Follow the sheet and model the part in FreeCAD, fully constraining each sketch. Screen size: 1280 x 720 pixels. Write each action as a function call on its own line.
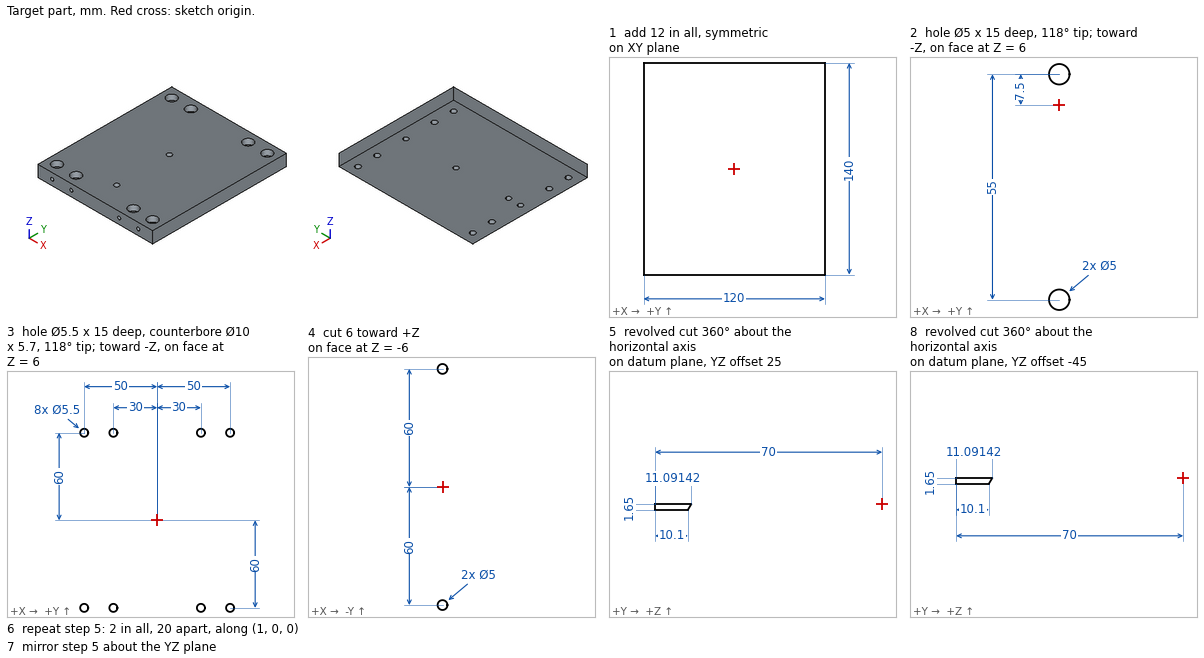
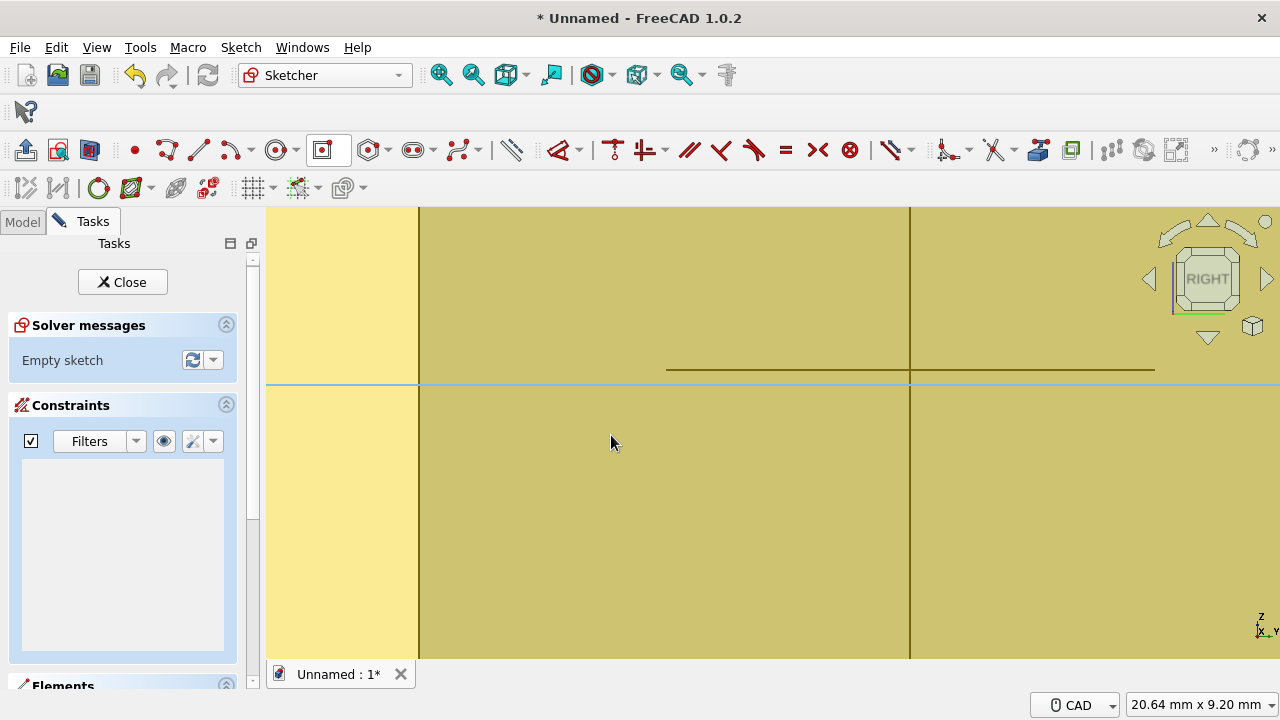
key(g)
key(m)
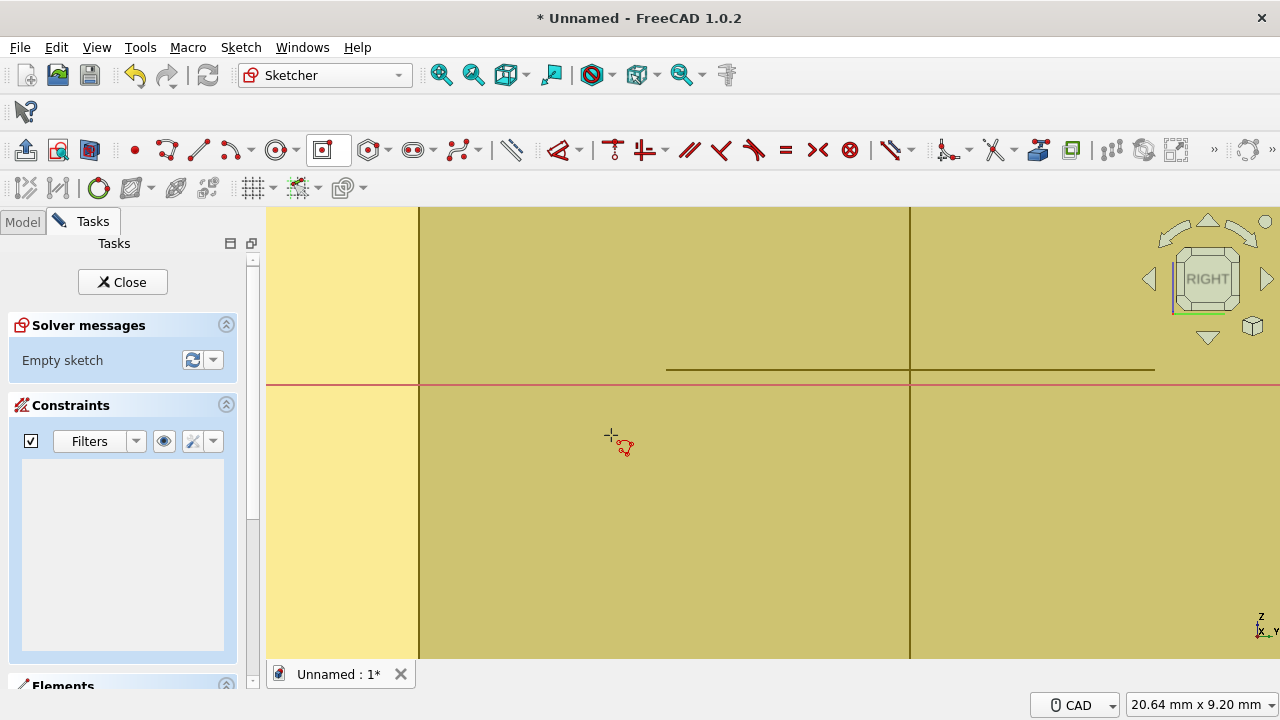
click(964, 385)
click(915, 466)
click(419, 466)
click(419, 394)
click(964, 385)
key(Escape)
key(Escape)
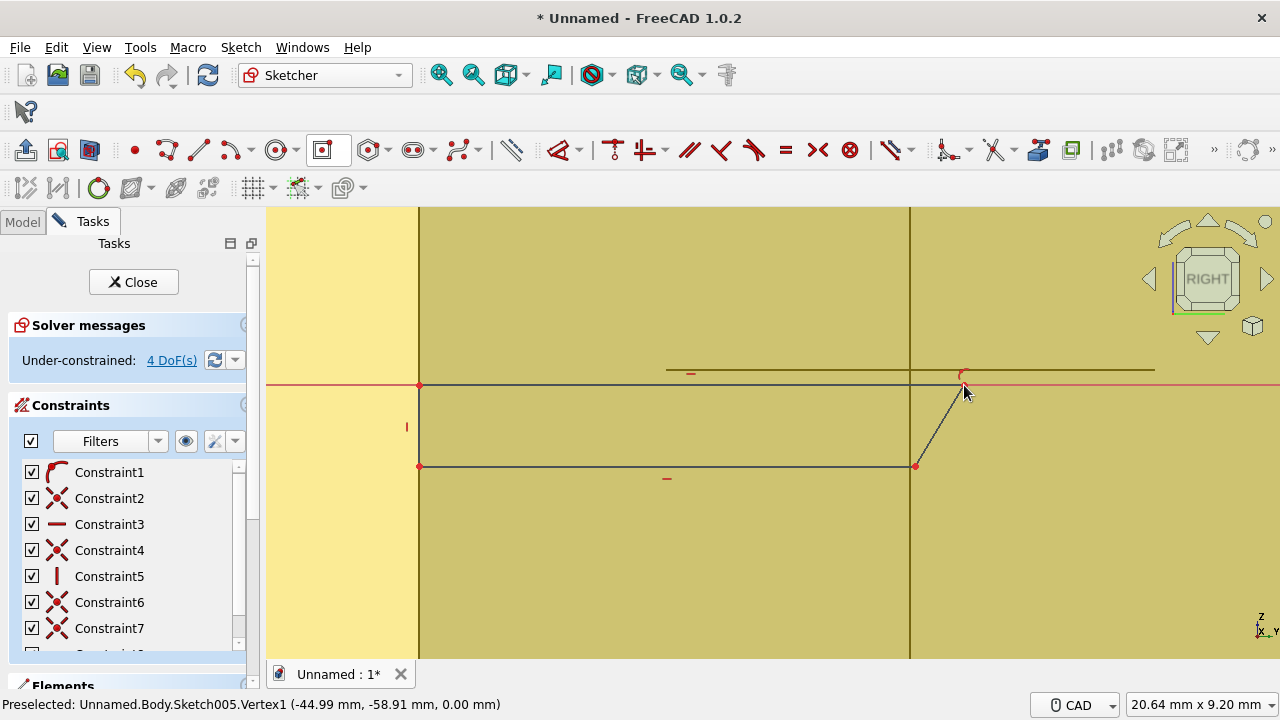
click(558, 150)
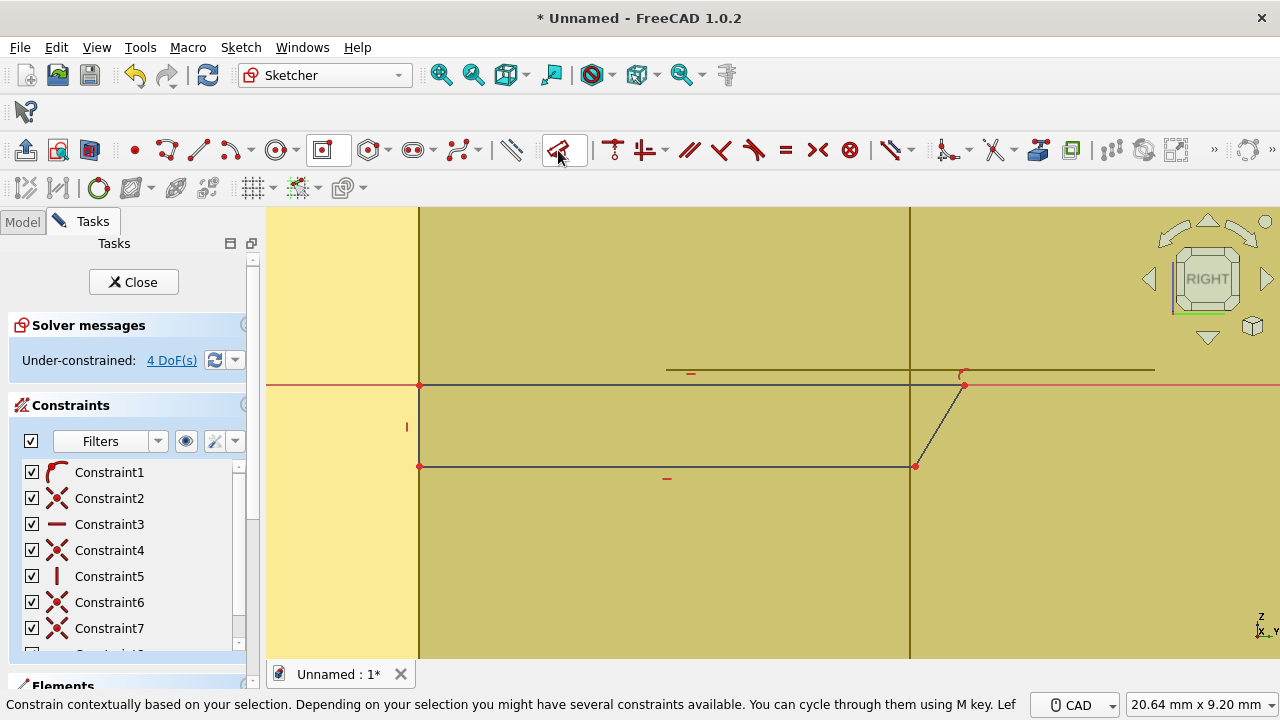
click(419, 467)
click(767, 501)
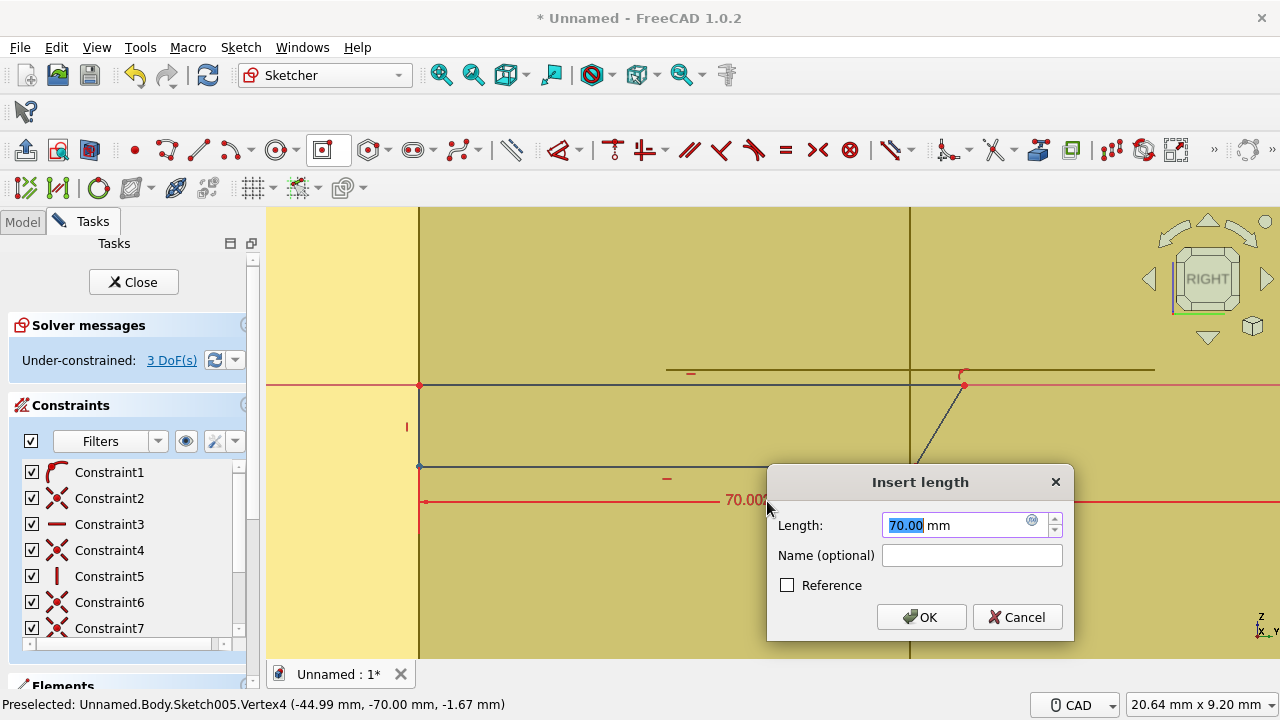
text(70)
key(Return)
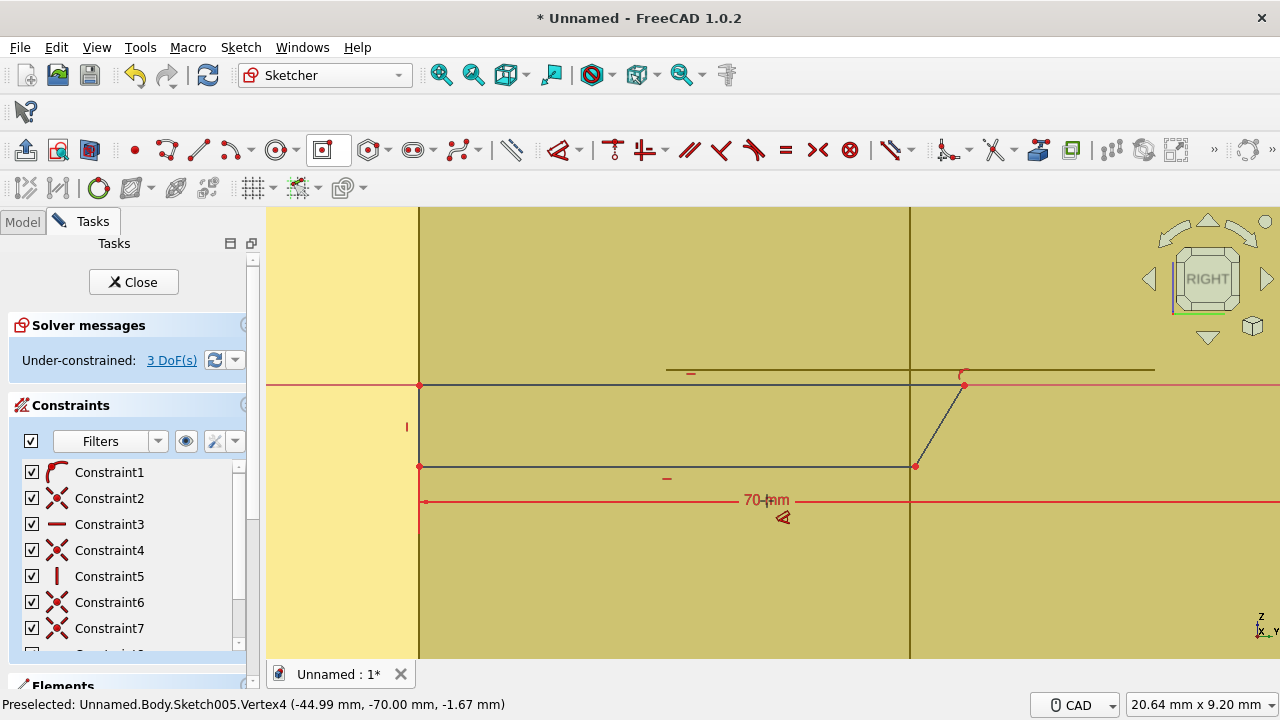
click(766, 467)
click(667, 501)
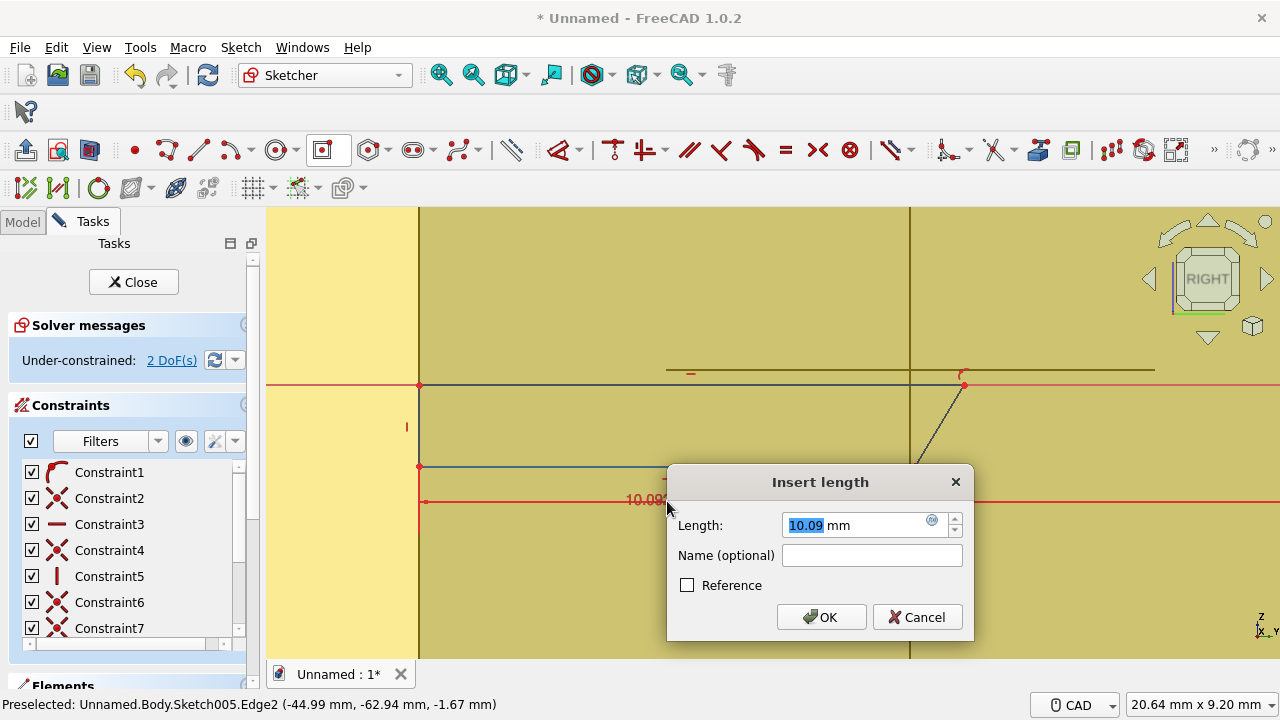
text(10.1)
key(Return)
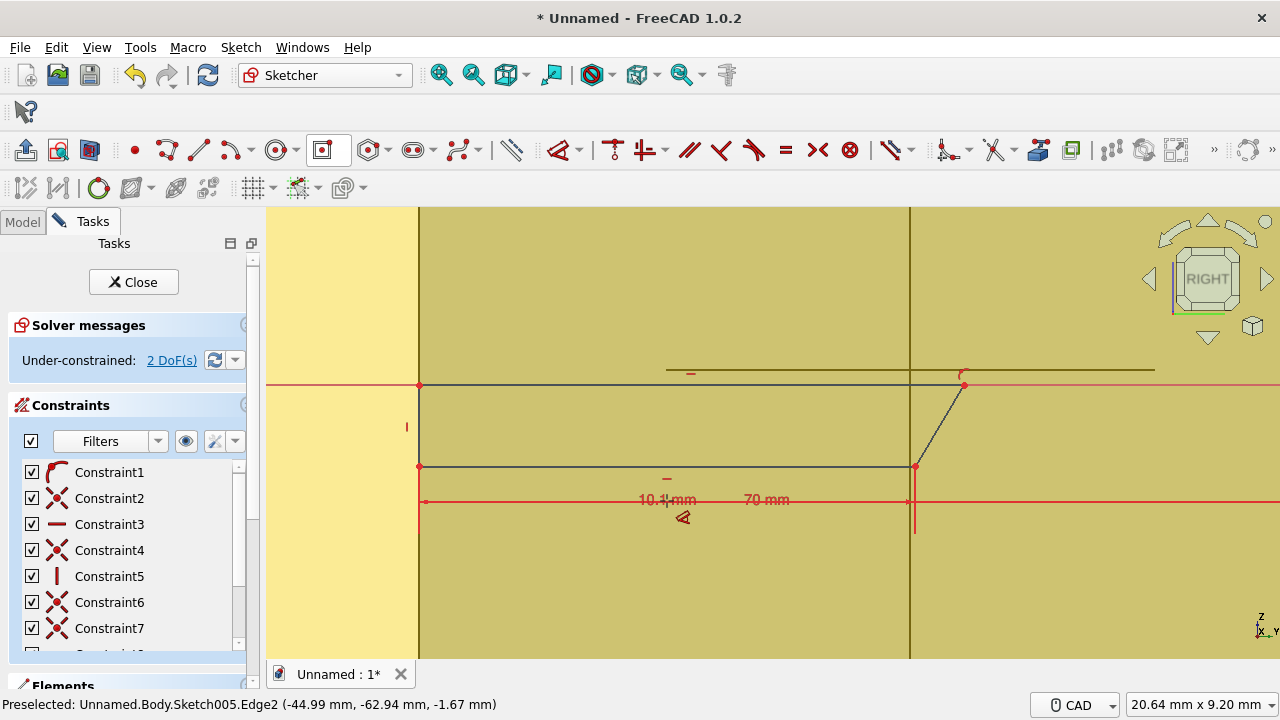
click(419, 442)
click(385, 426)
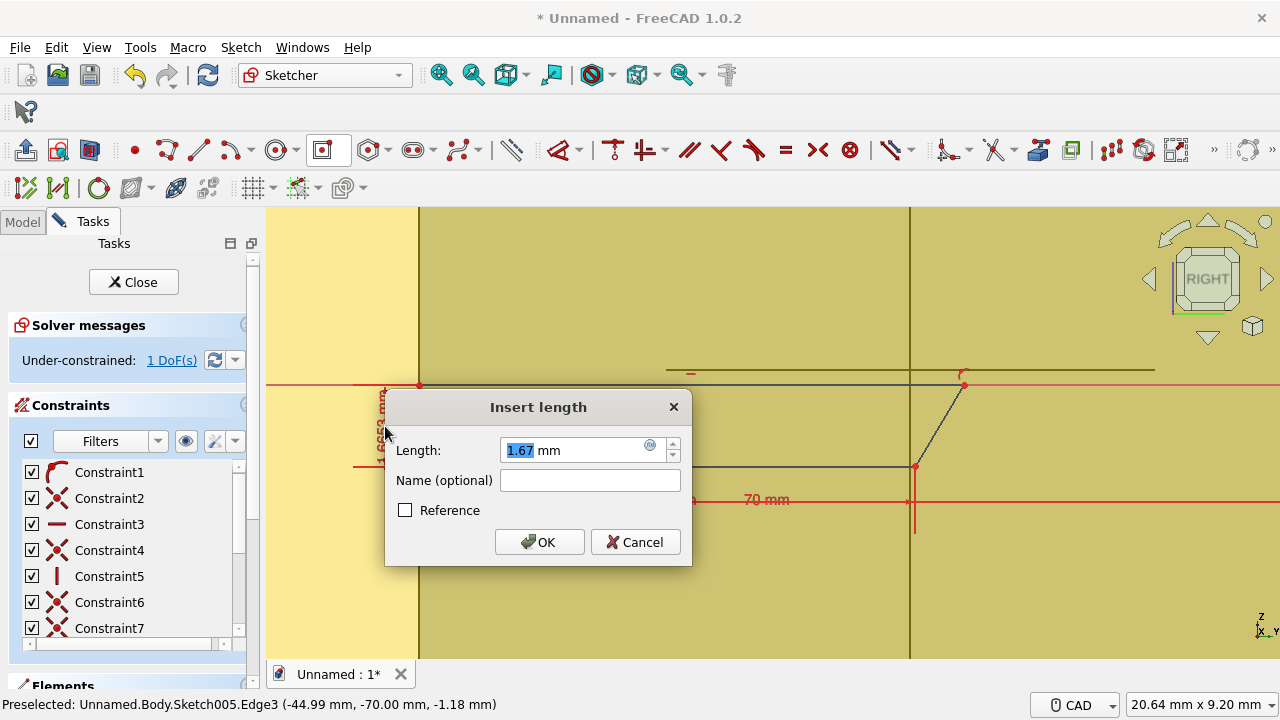
text(1.65)
key(Return)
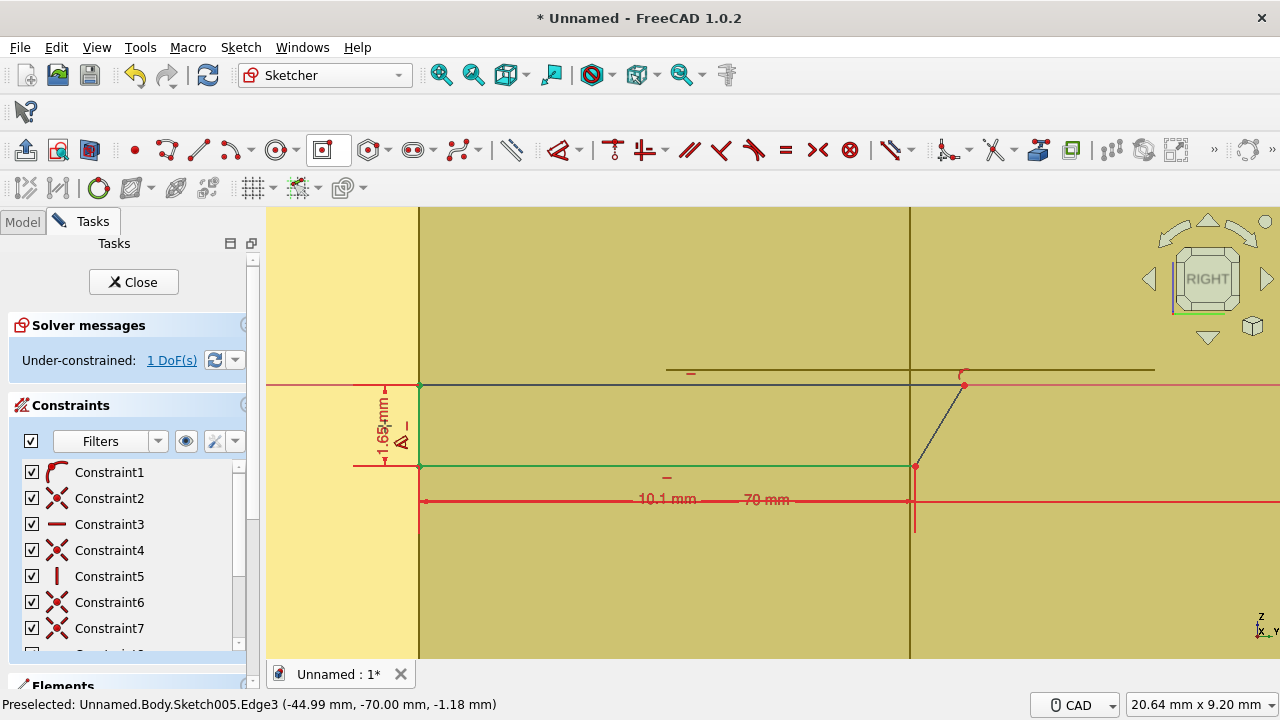
click(583, 385)
click(692, 351)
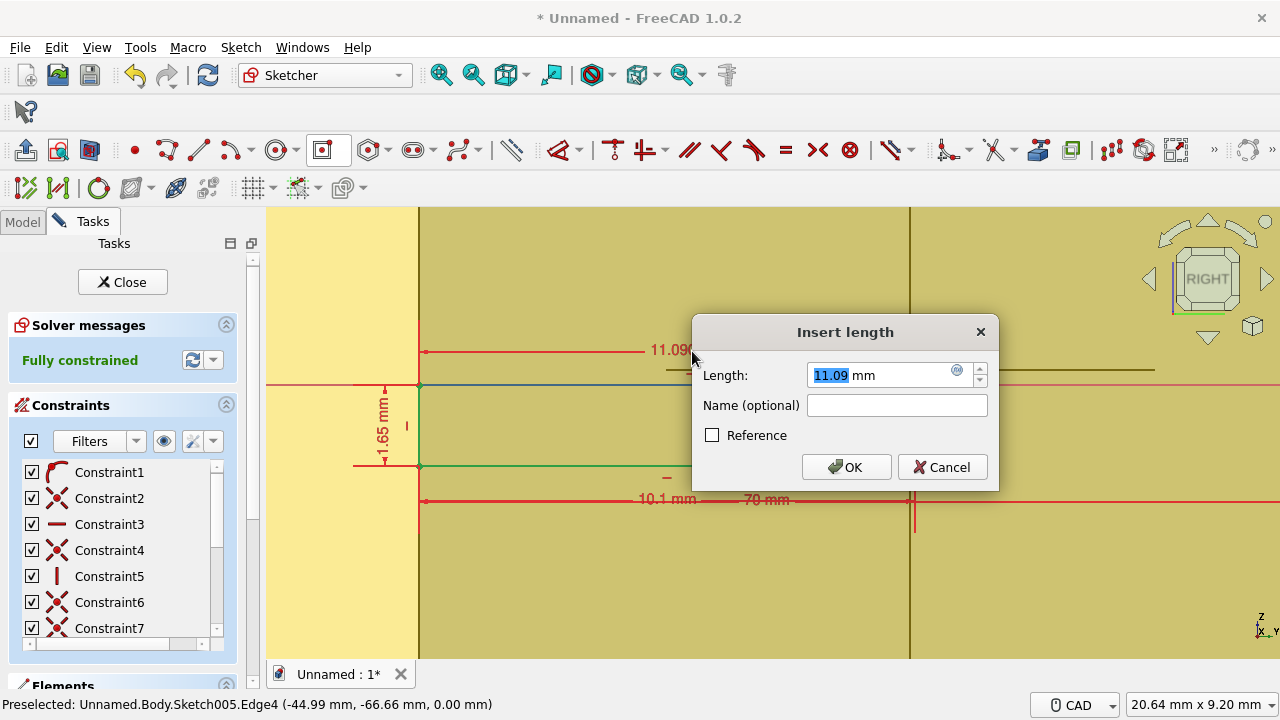
text(11.09142)
key(Return)
key(Escape)